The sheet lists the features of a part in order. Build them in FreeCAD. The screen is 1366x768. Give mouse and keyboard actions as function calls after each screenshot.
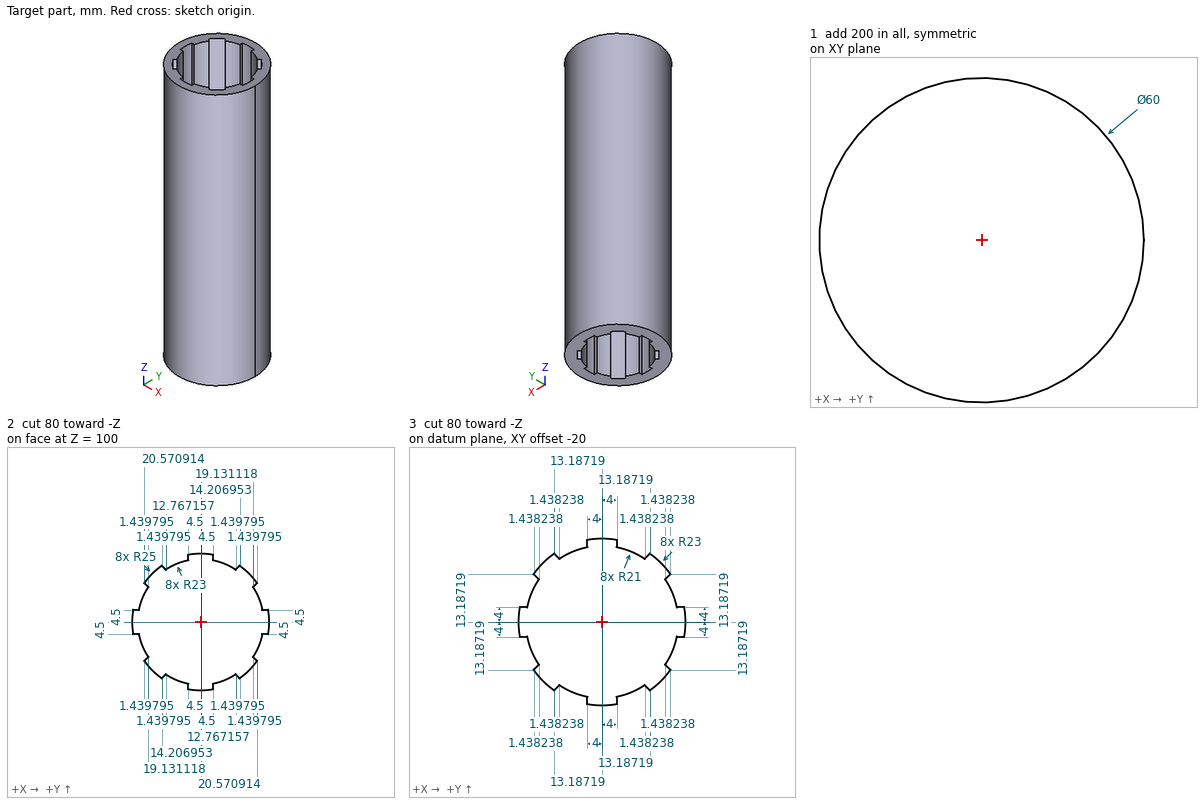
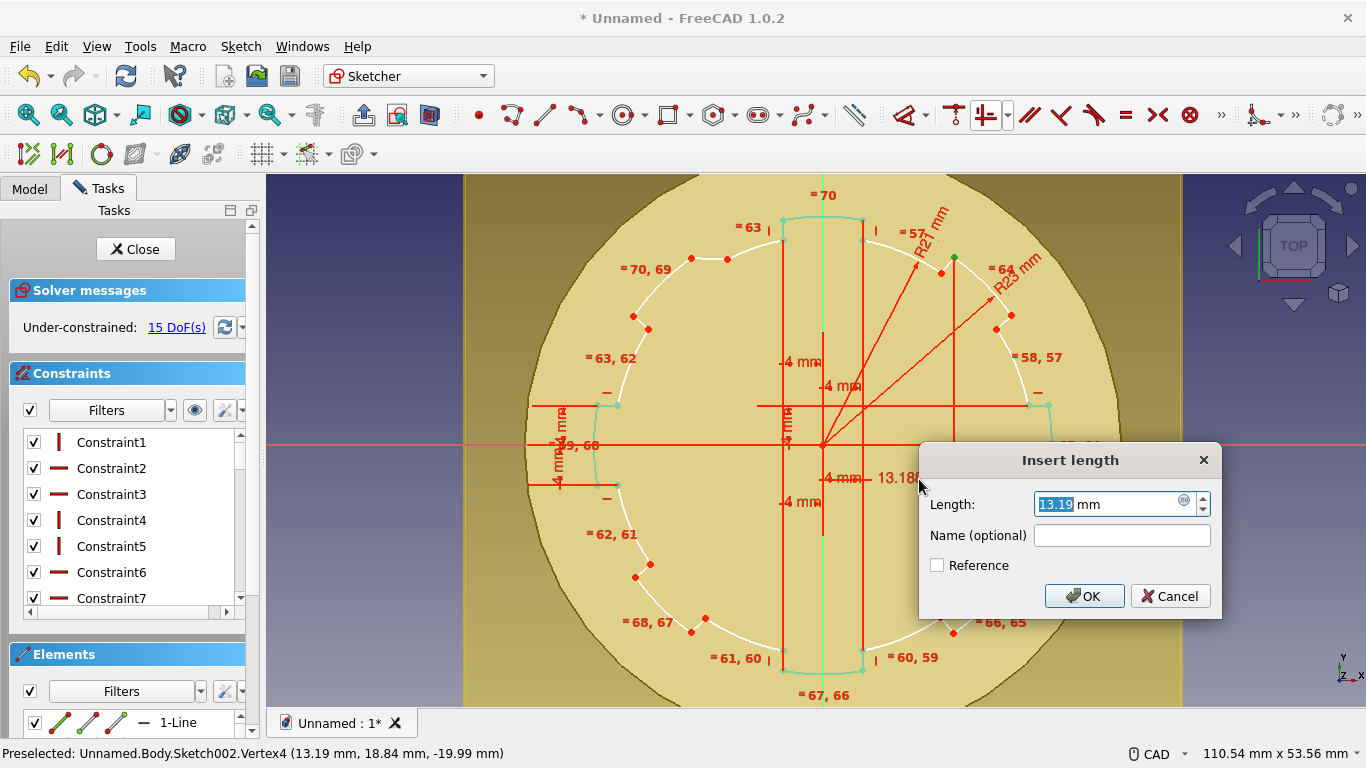
text(13.18719)
key(Return)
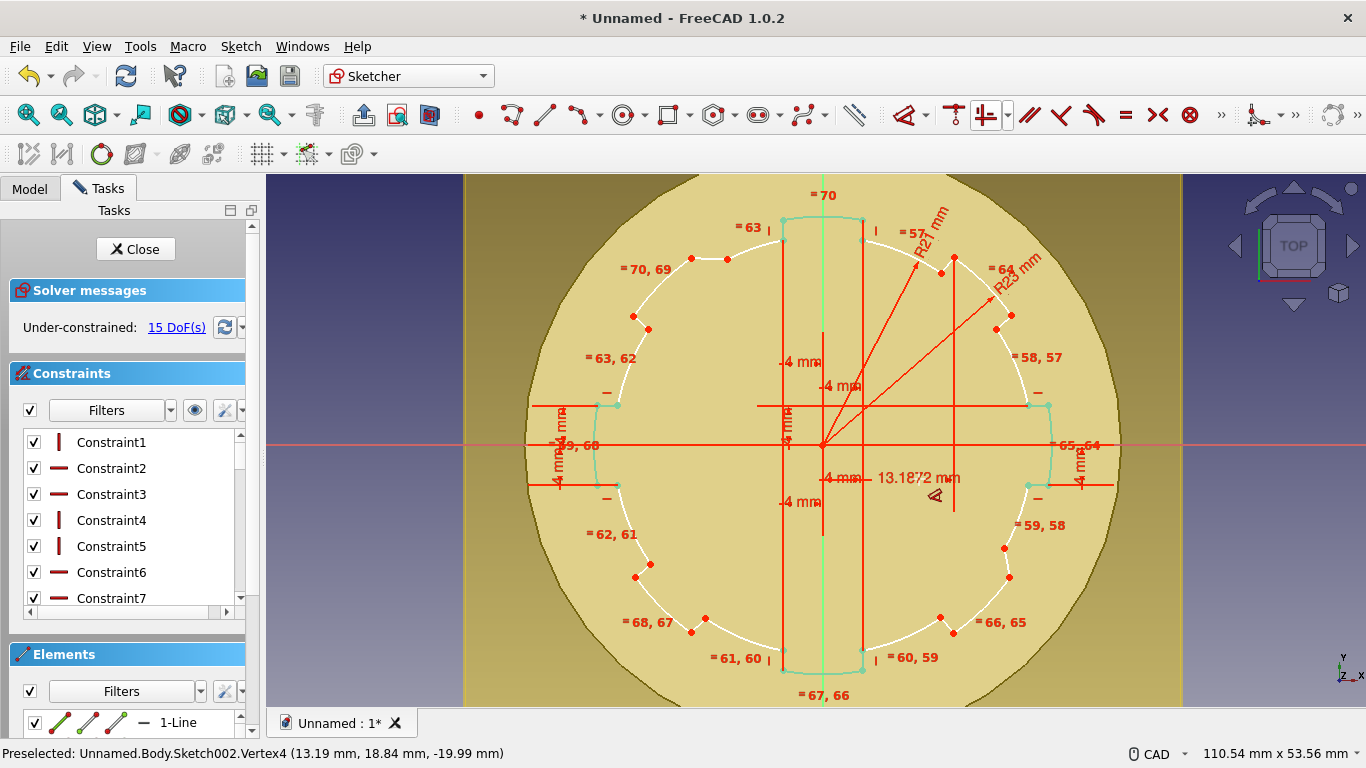
click(1012, 316)
click(1046, 381)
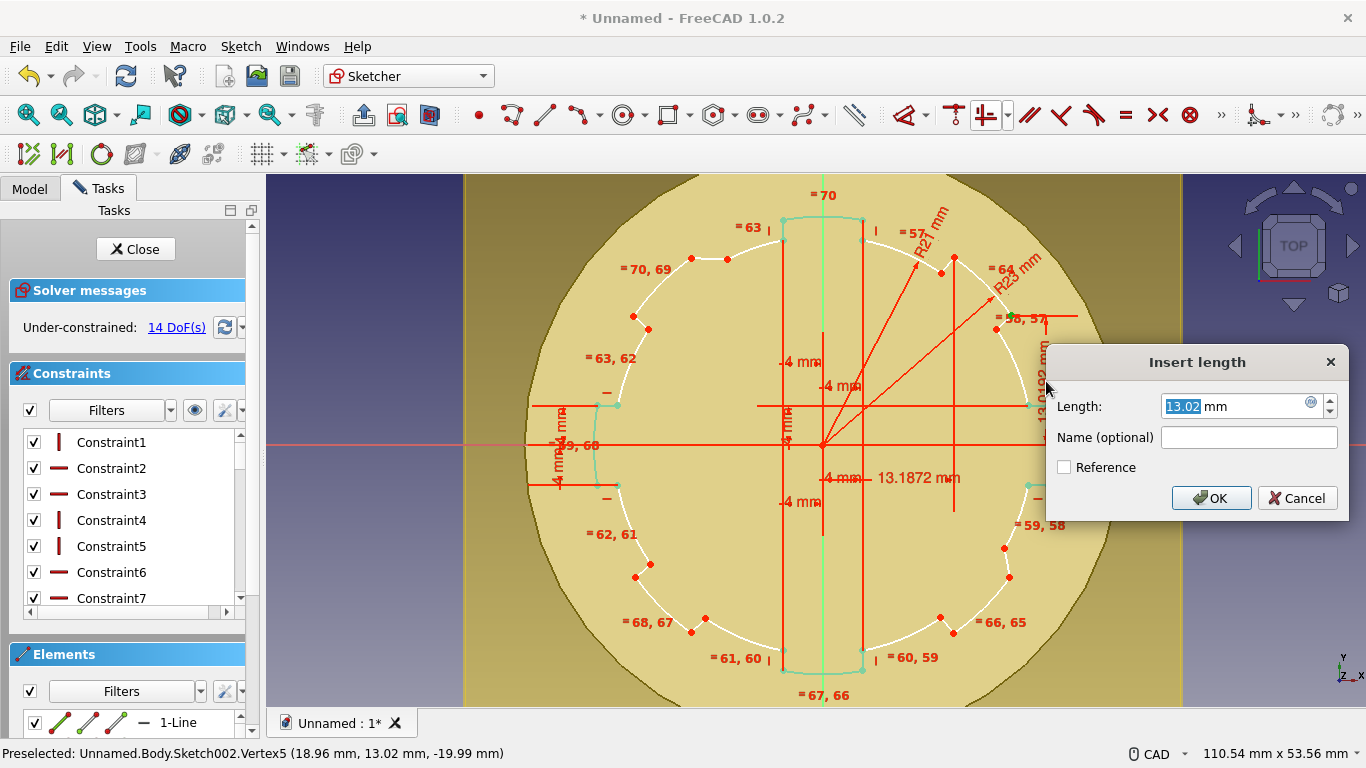
text(13.18719)
key(Return)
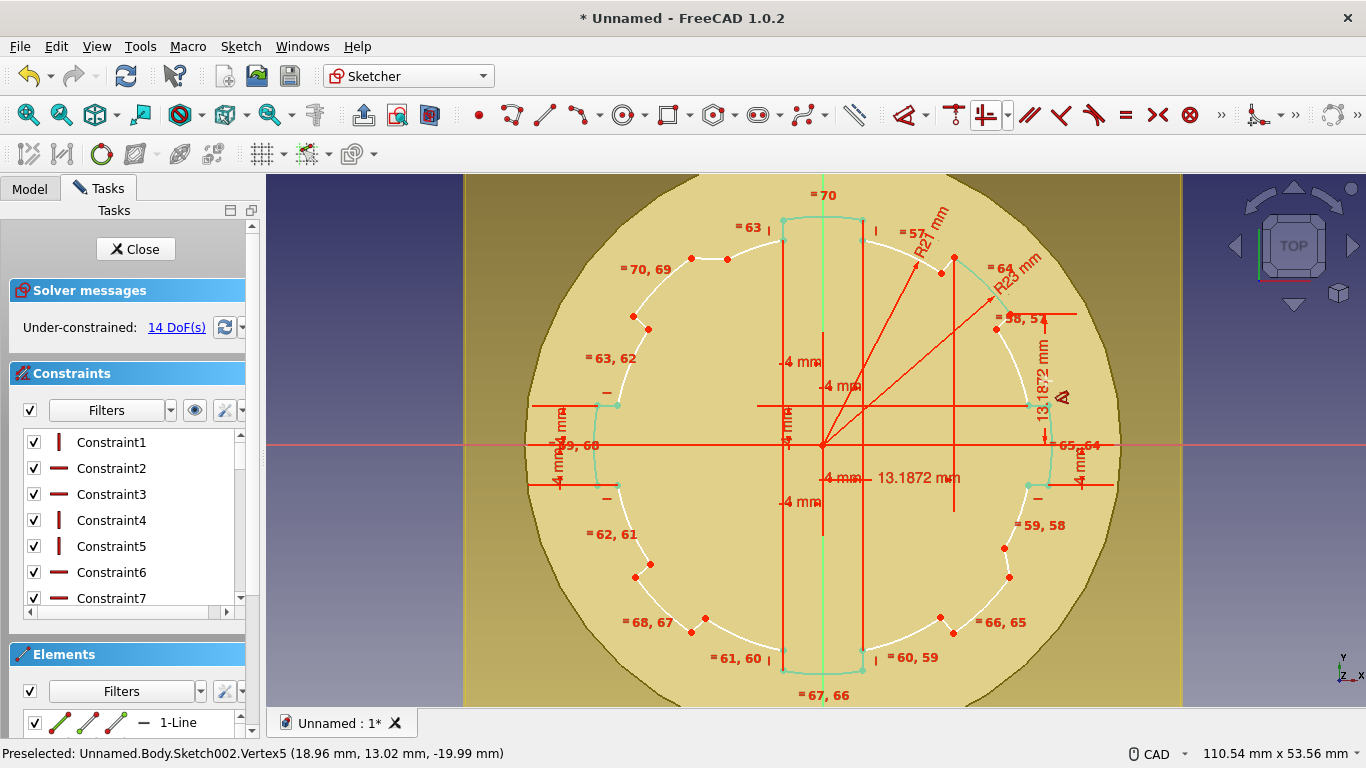
click(1010, 577)
click(1044, 511)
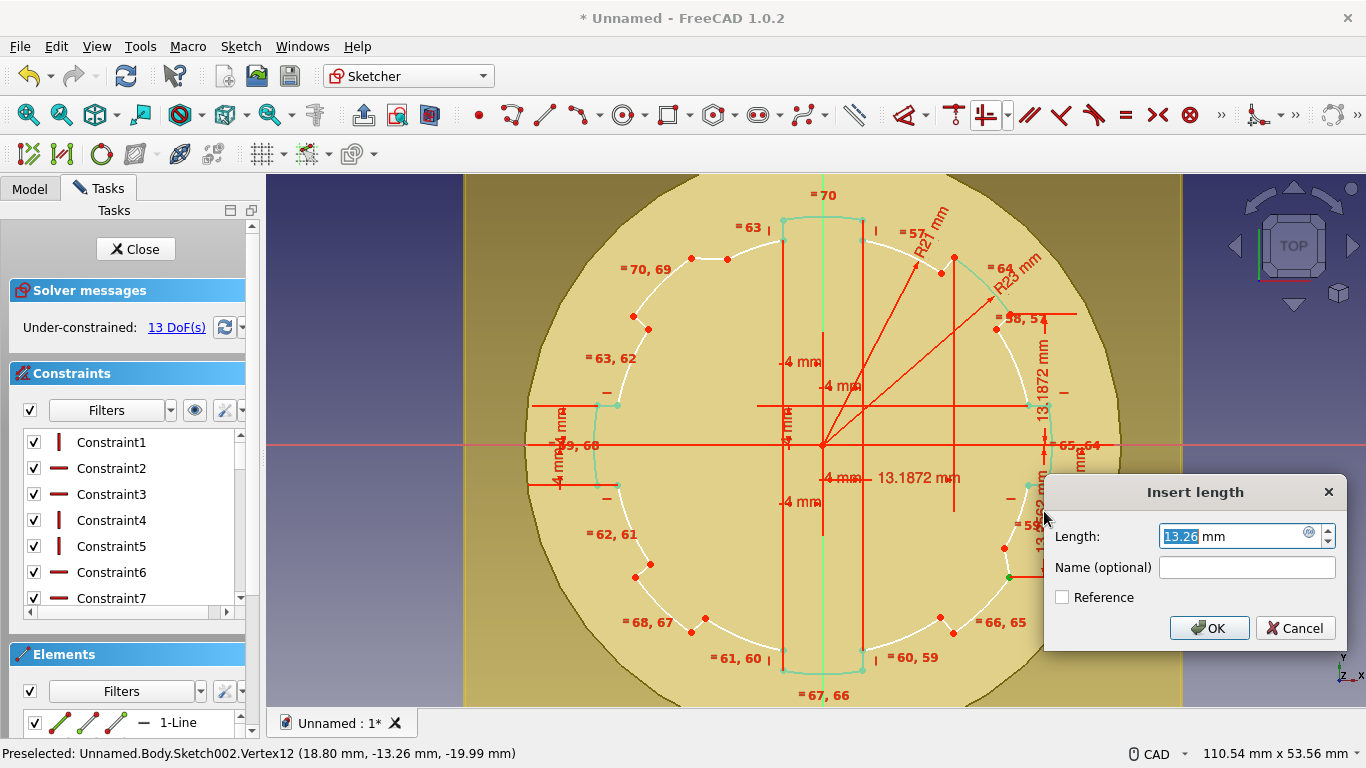
text(13.18719)
key(Return)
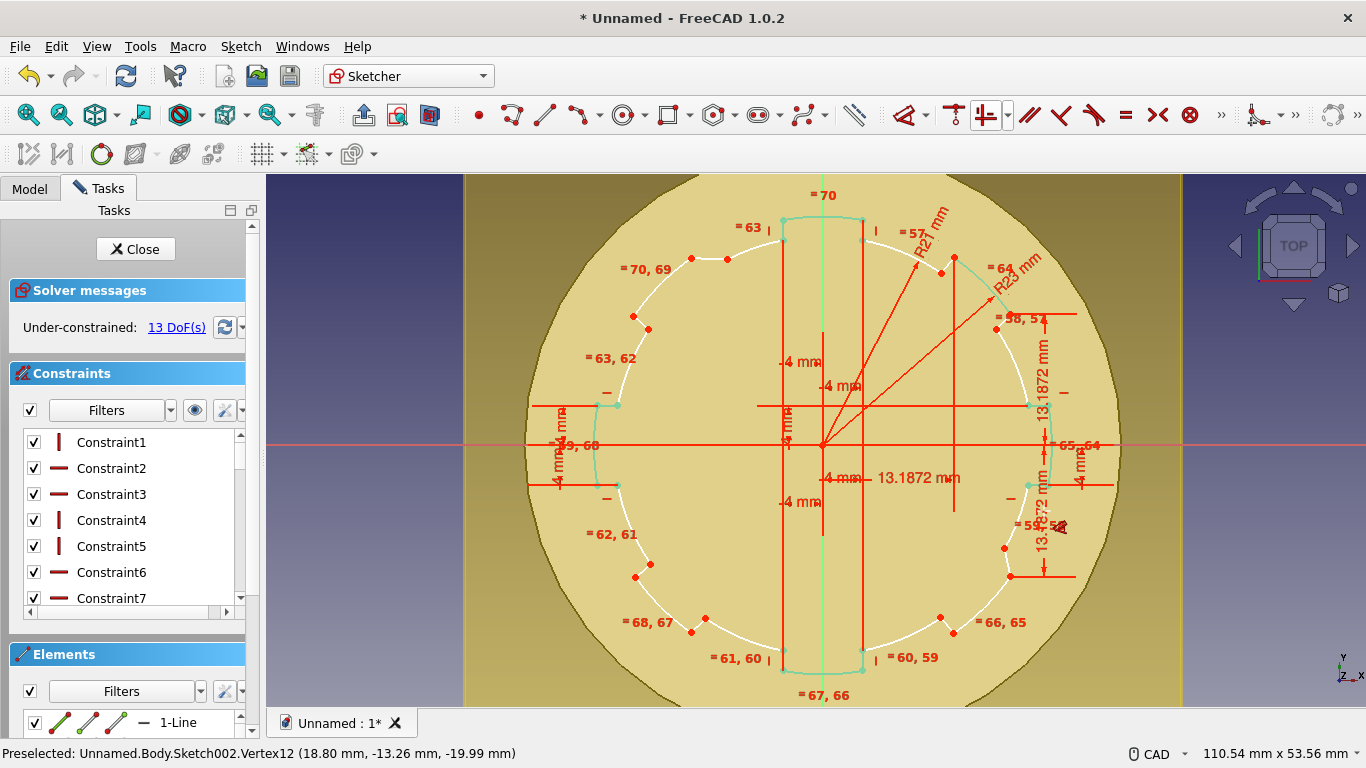
click(954, 633)
click(888, 667)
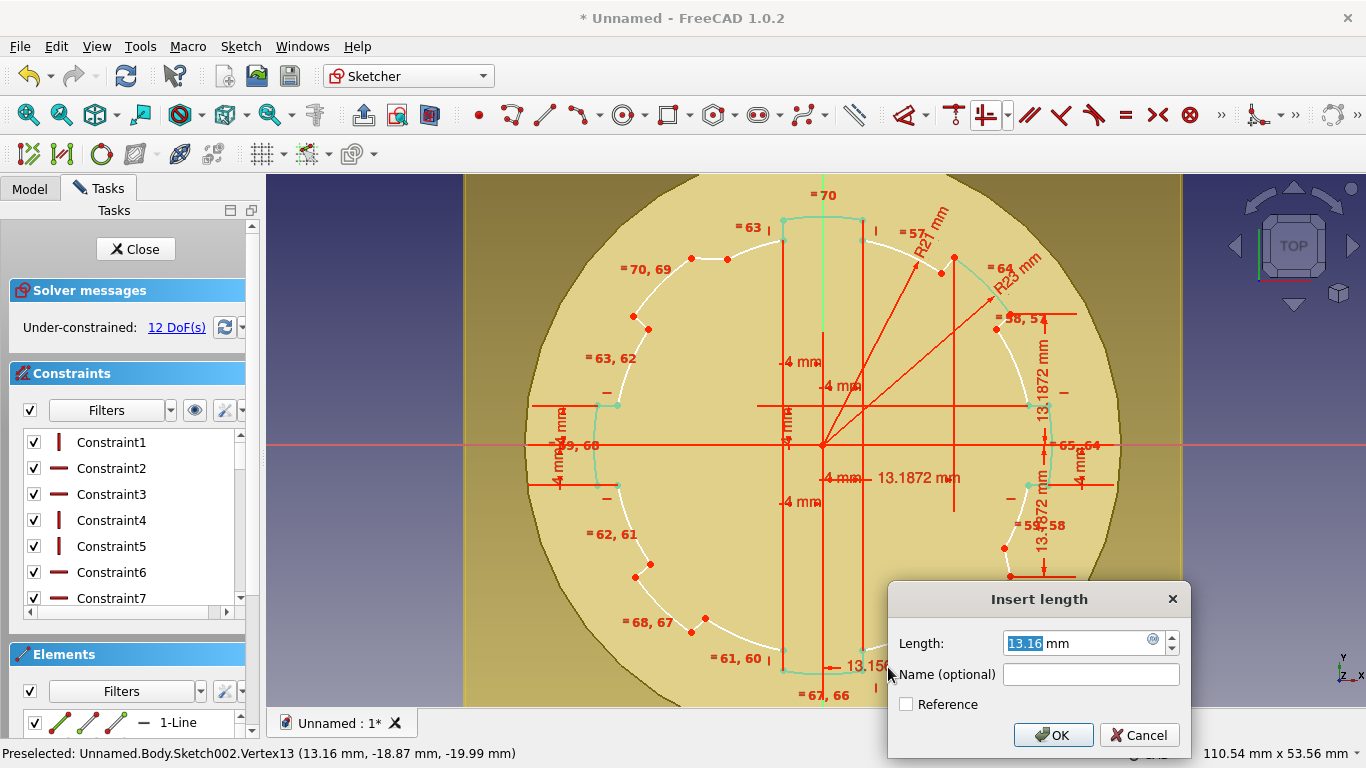
text(13.18719)
key(Return)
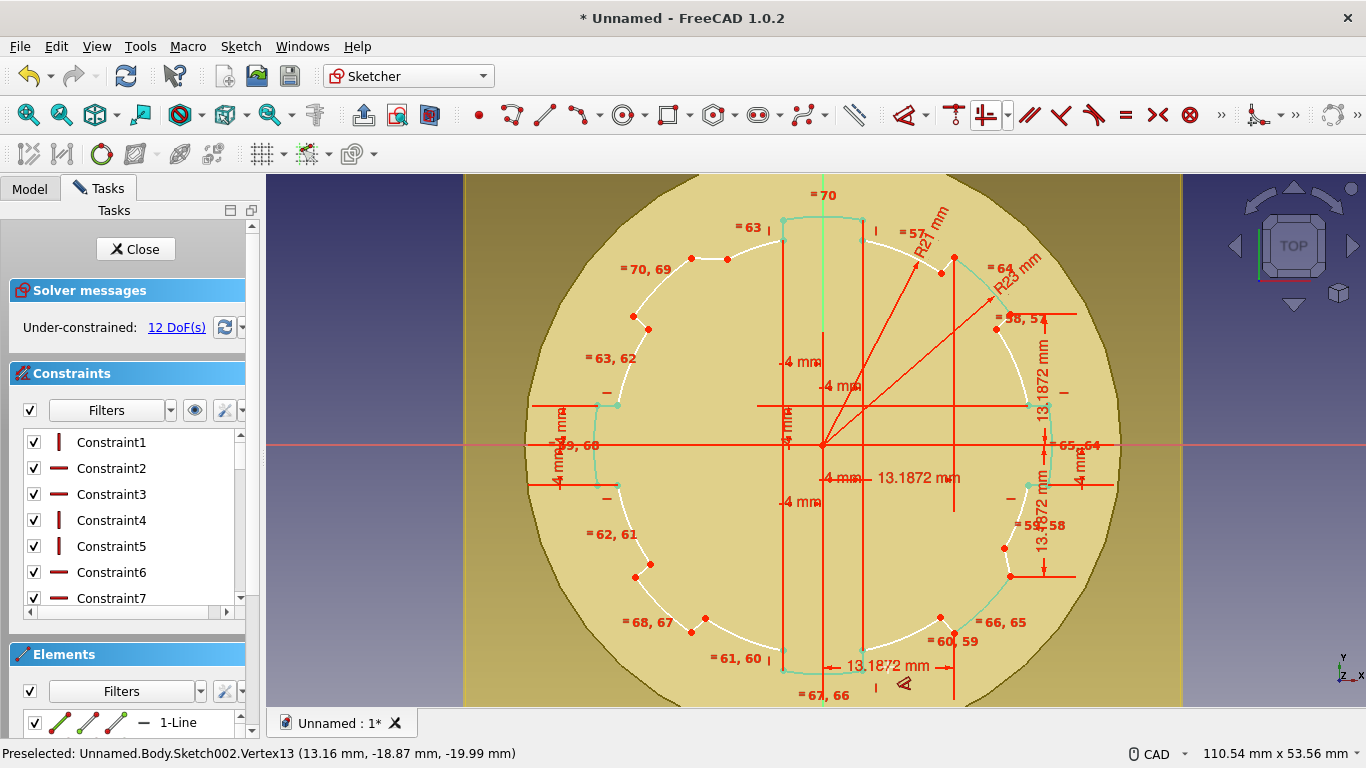
click(691, 633)
click(757, 667)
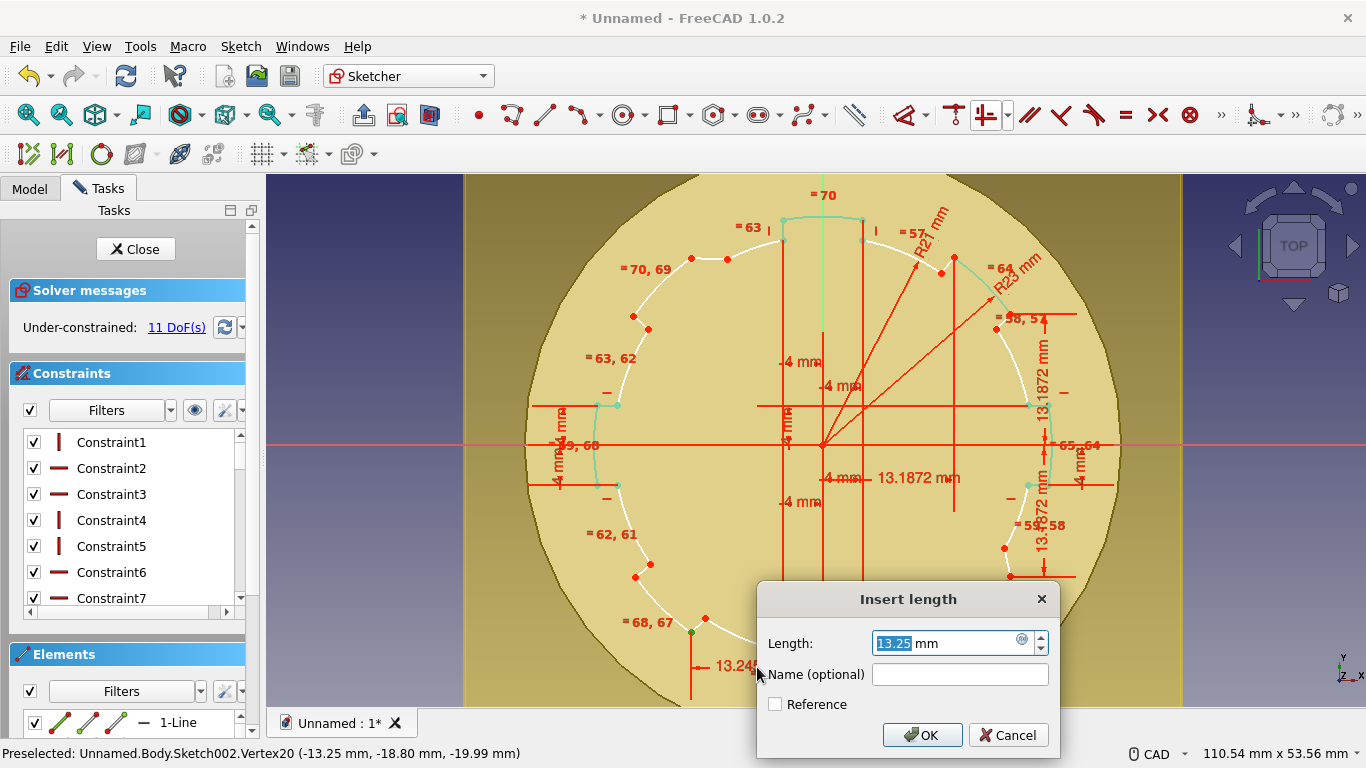
text(13.18719)
key(Return)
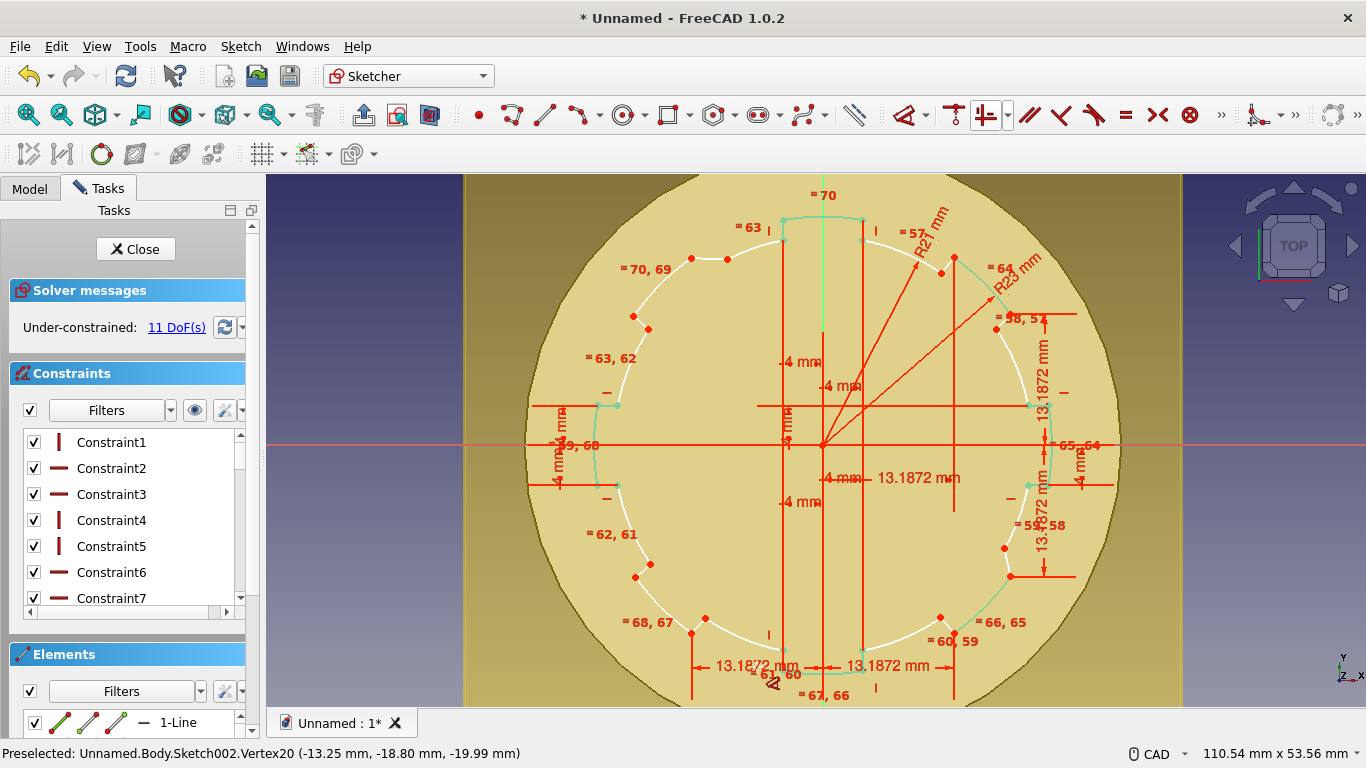
click(636, 577)
click(602, 511)